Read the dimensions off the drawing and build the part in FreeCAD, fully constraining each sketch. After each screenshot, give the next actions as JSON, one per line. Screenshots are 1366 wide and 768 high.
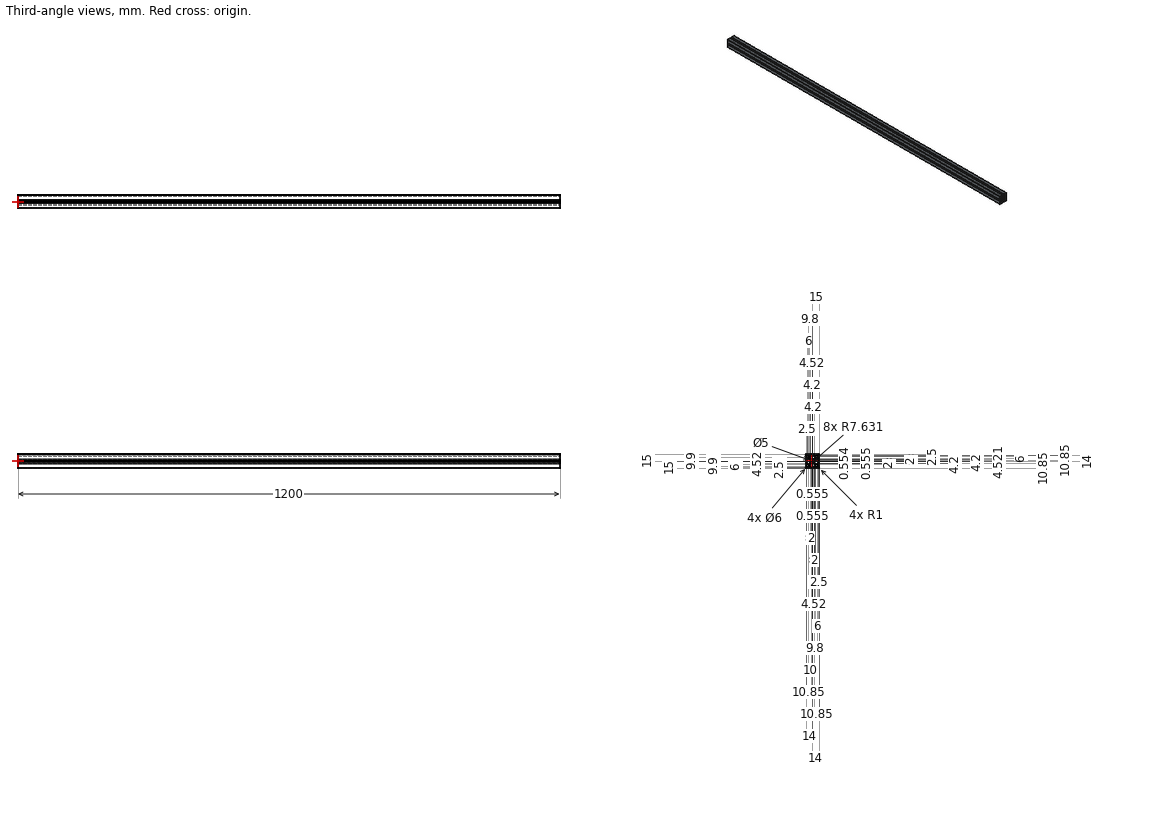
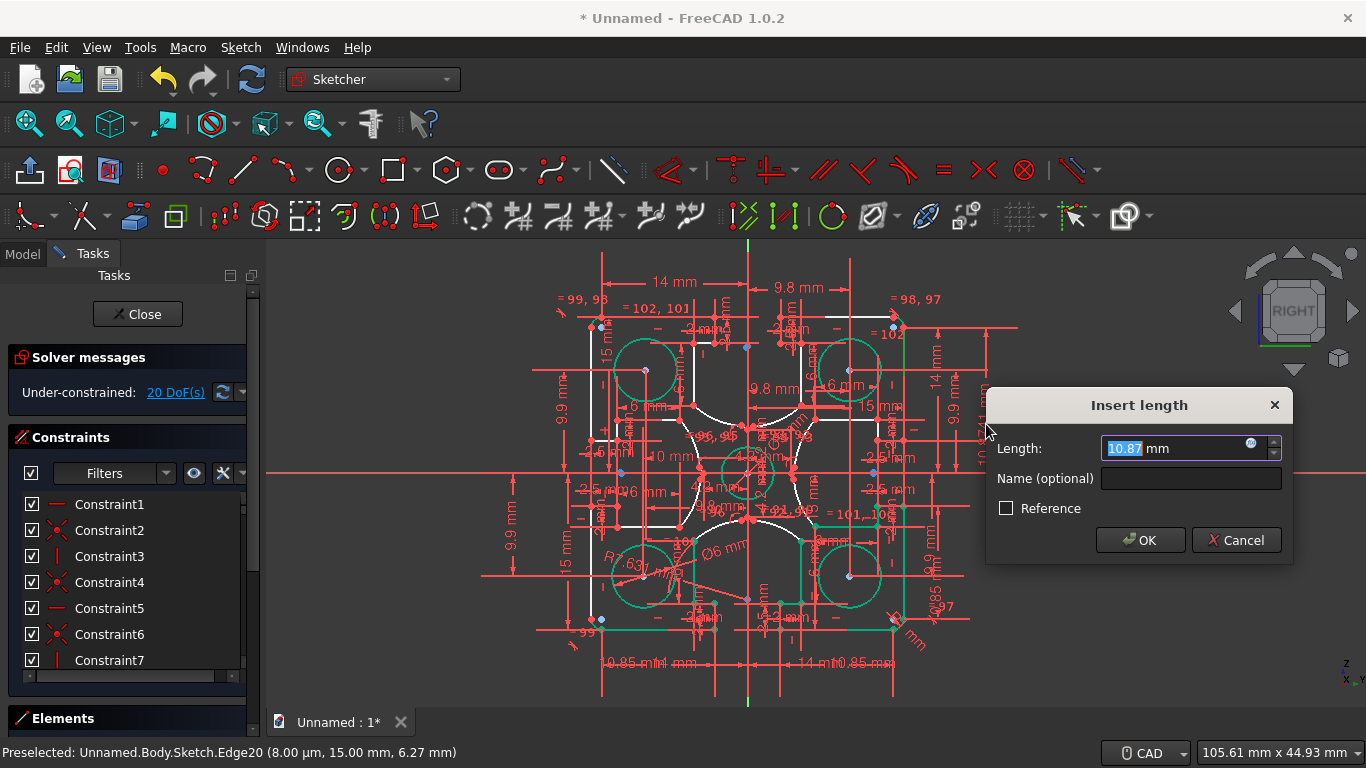
{"action": "type", "text": "10.85"}
{"action": "key", "text": "Return"}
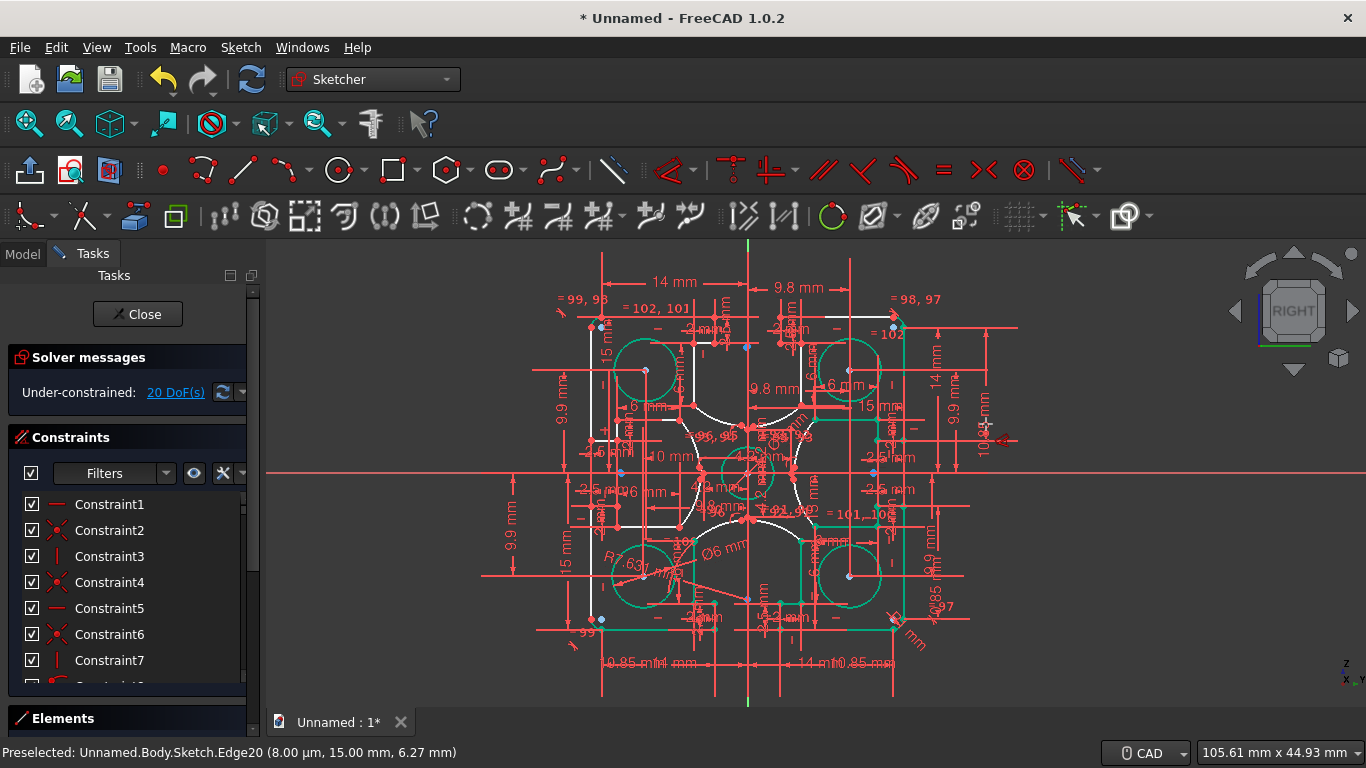
{"action": "left_click", "coordinate": [860, 317]}
{"action": "left_click", "coordinate": [877, 283]}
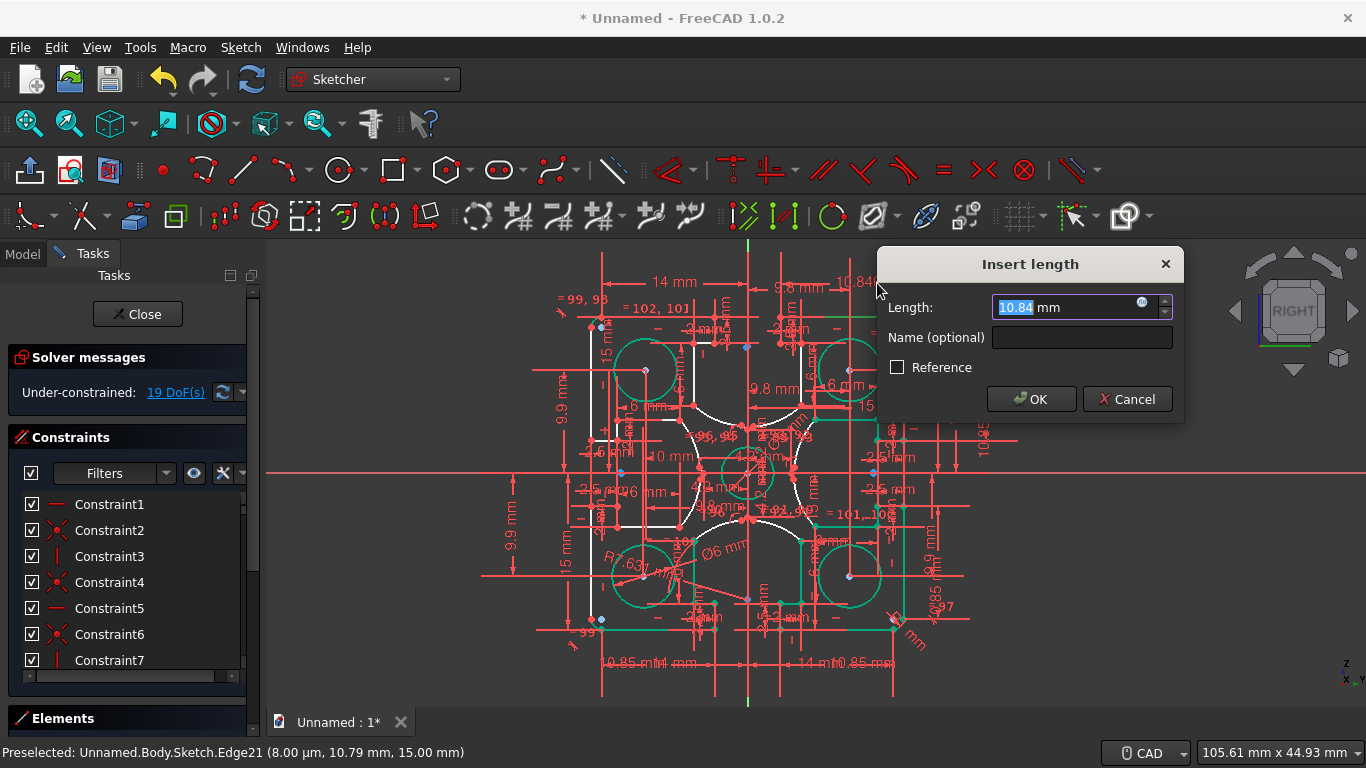
{"action": "type", "text": "10.85"}
{"action": "key", "text": "Return"}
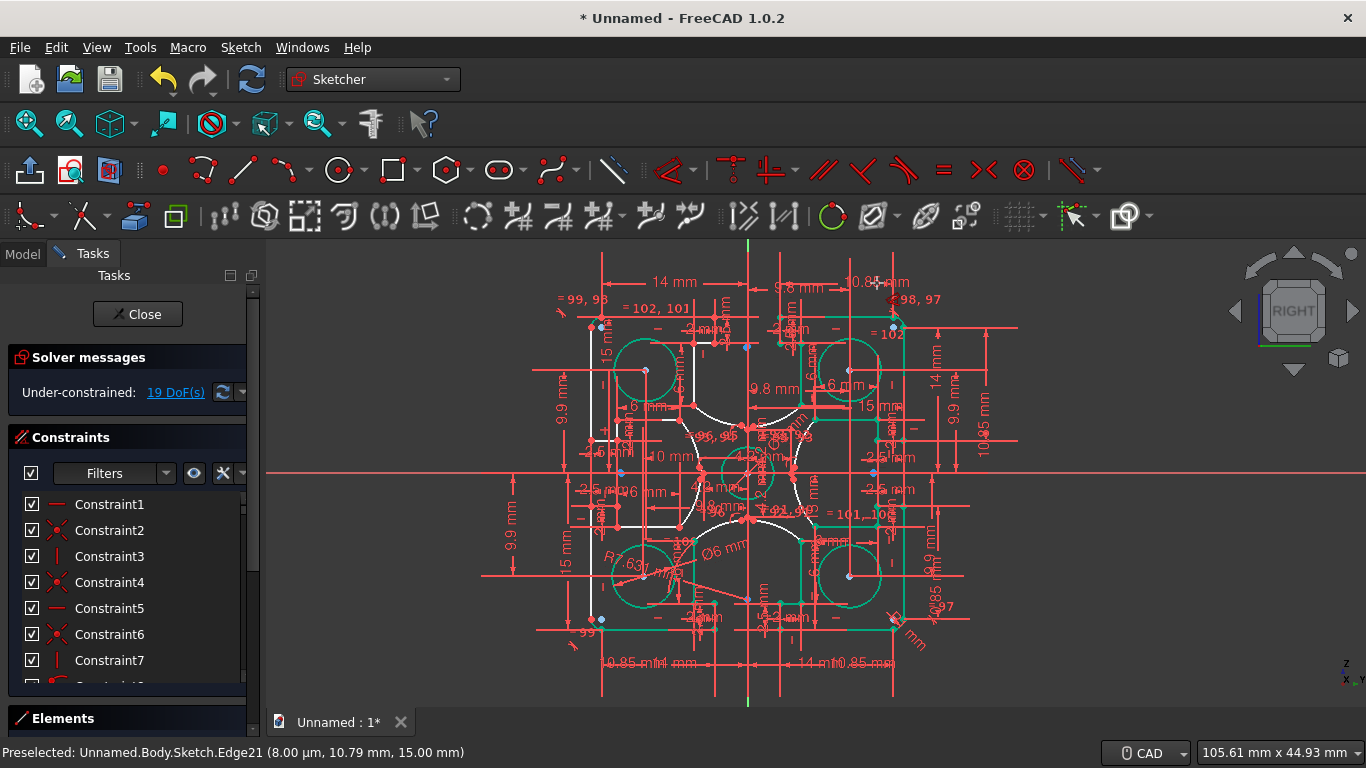
{"action": "left_click", "coordinate": [681, 317]}
{"action": "left_click", "coordinate": [632, 283]}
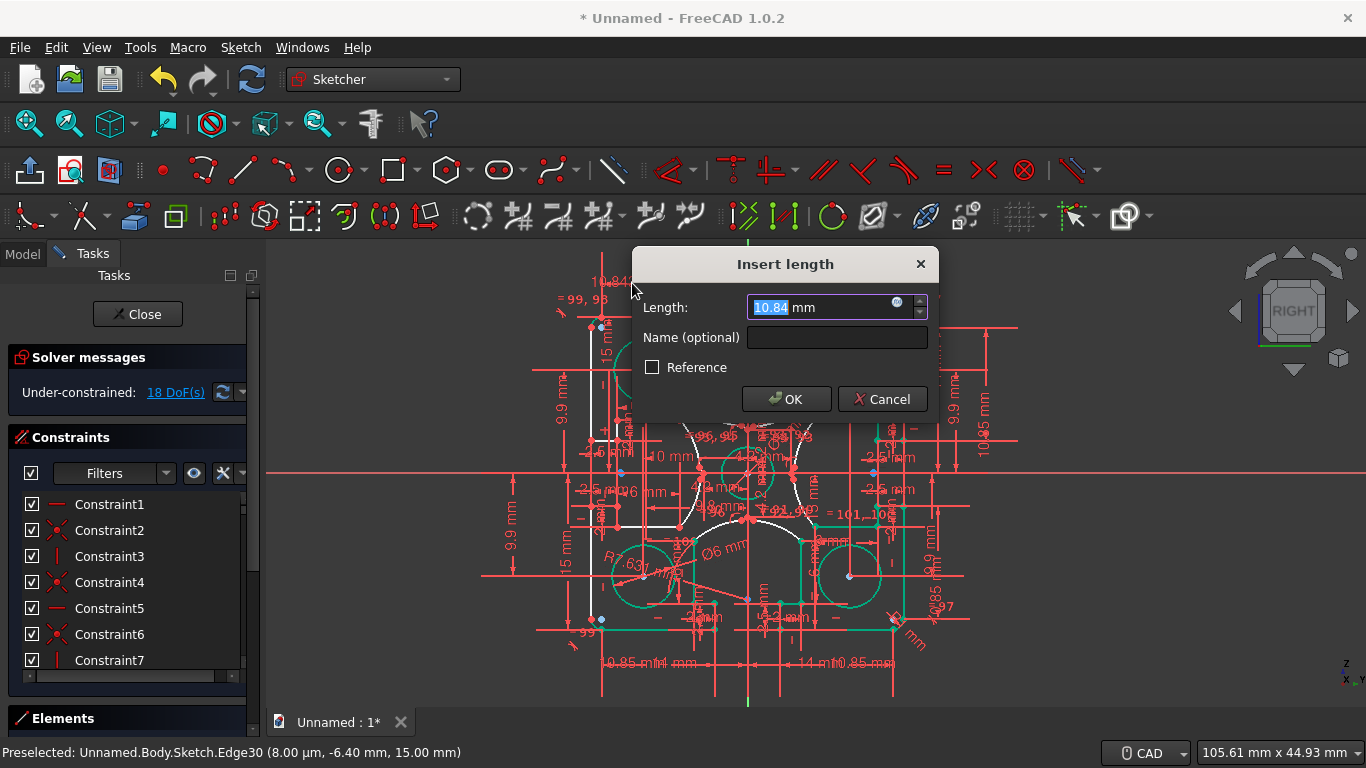
{"action": "type", "text": "10.85"}
{"action": "key", "text": "Return"}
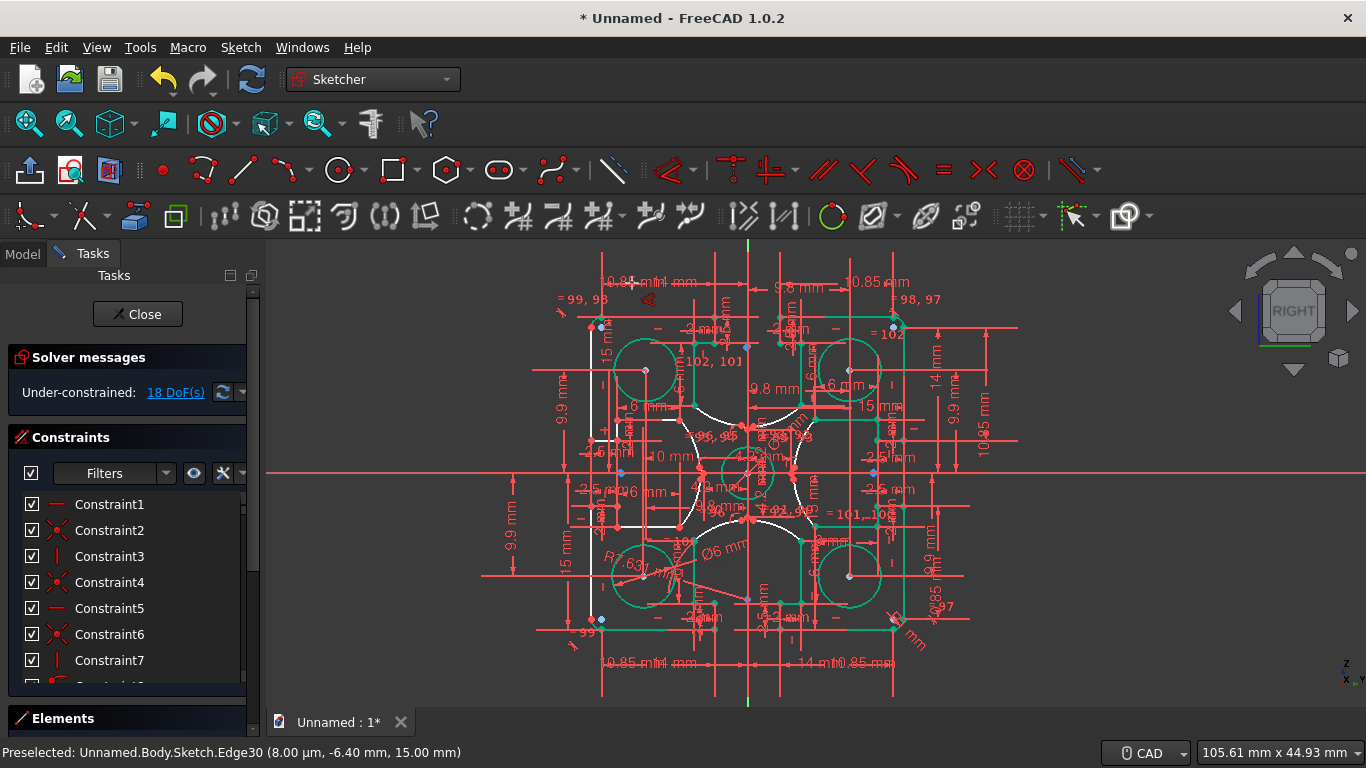
{"action": "left_click", "coordinate": [591, 362]}
{"action": "left_click", "coordinate": [557, 424]}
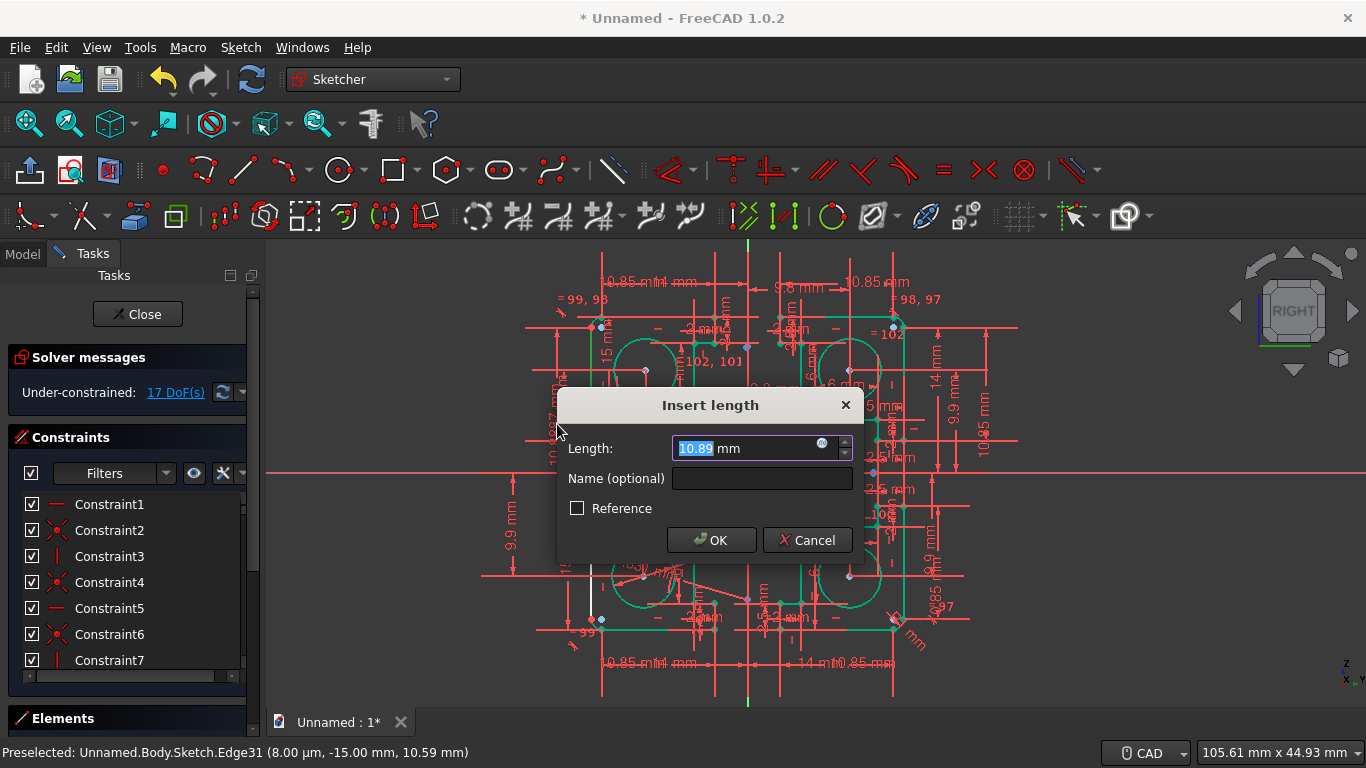
{"action": "type", "text": "10.85"}
{"action": "key", "text": "Return"}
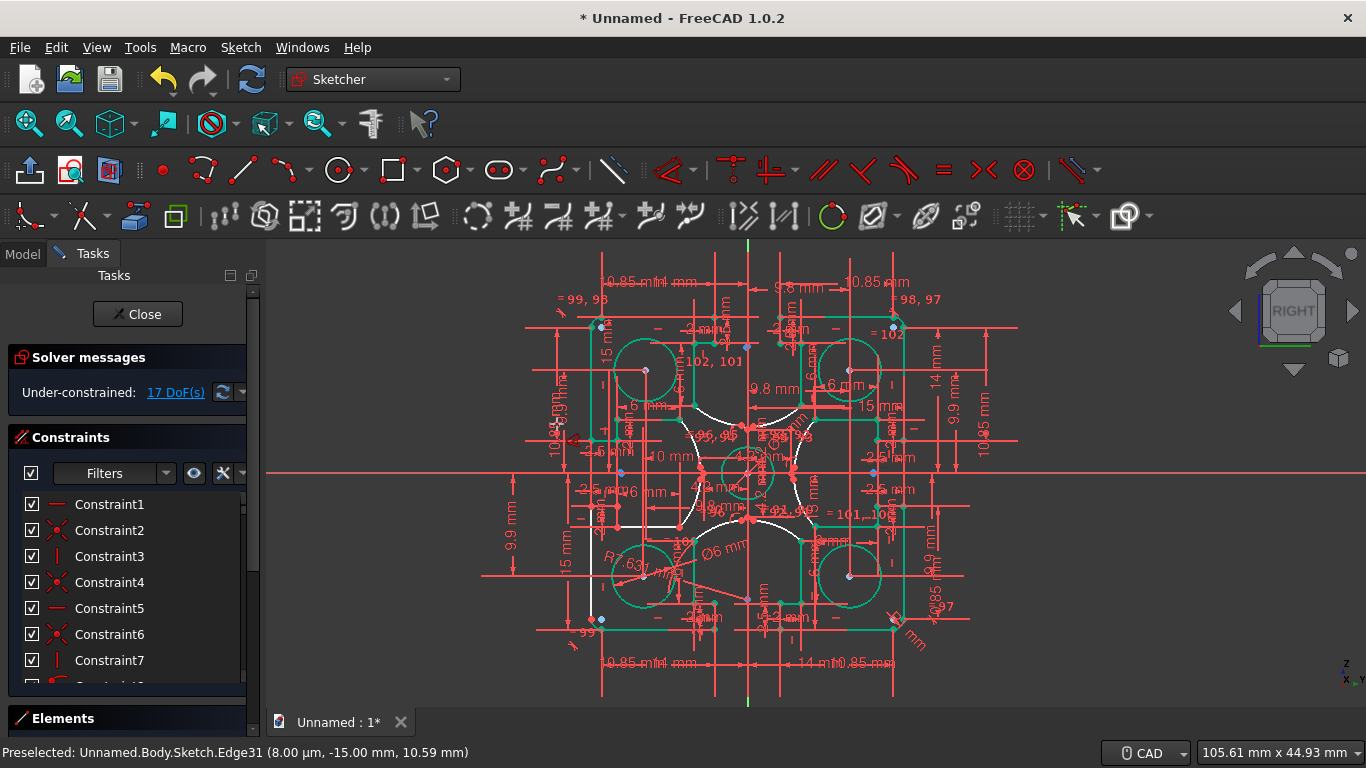
{"action": "left_click", "coordinate": [591, 540]}
{"action": "left_click", "coordinate": [557, 589]}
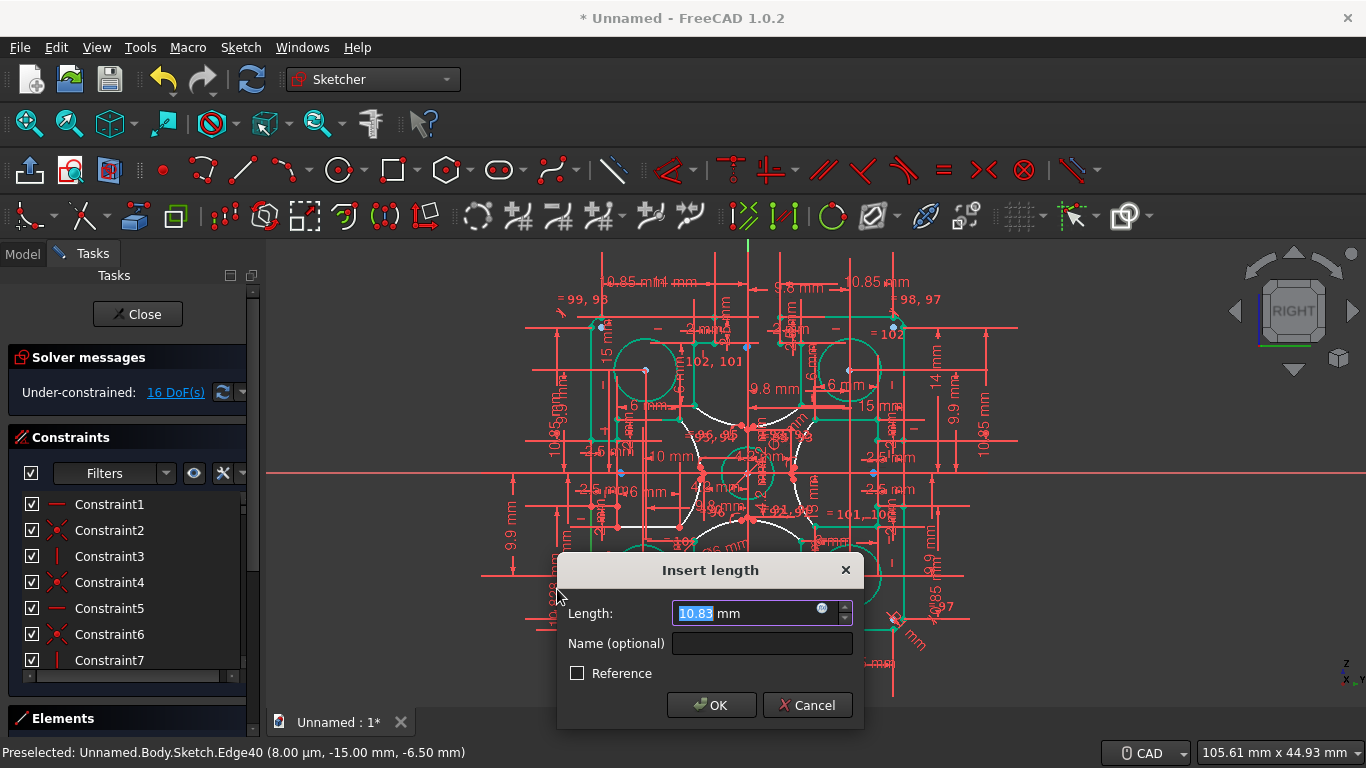
{"action": "type", "text": "10.85"}
{"action": "key", "text": "Return"}